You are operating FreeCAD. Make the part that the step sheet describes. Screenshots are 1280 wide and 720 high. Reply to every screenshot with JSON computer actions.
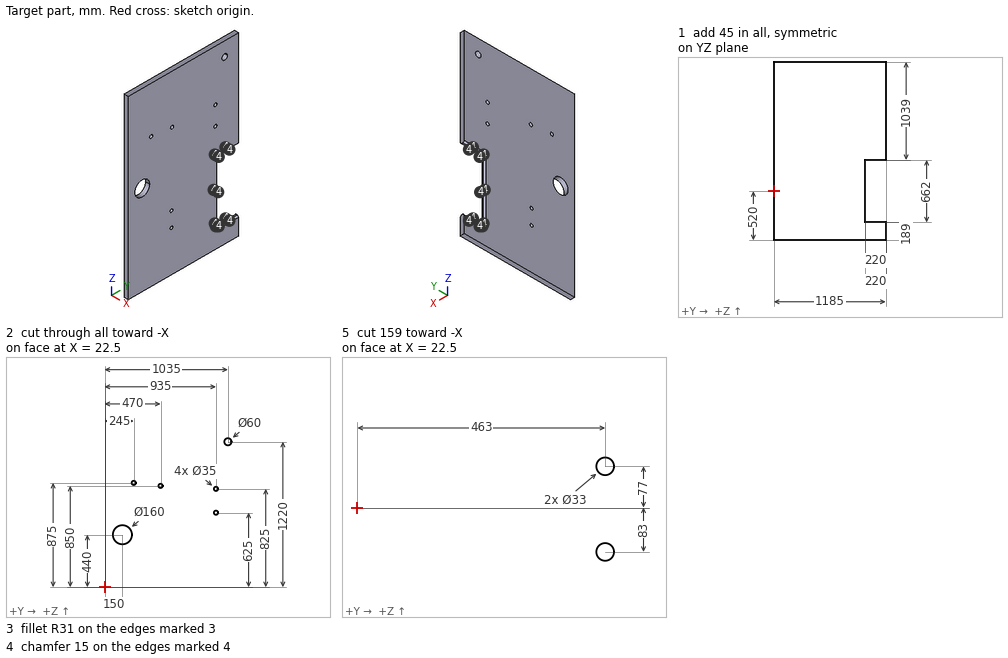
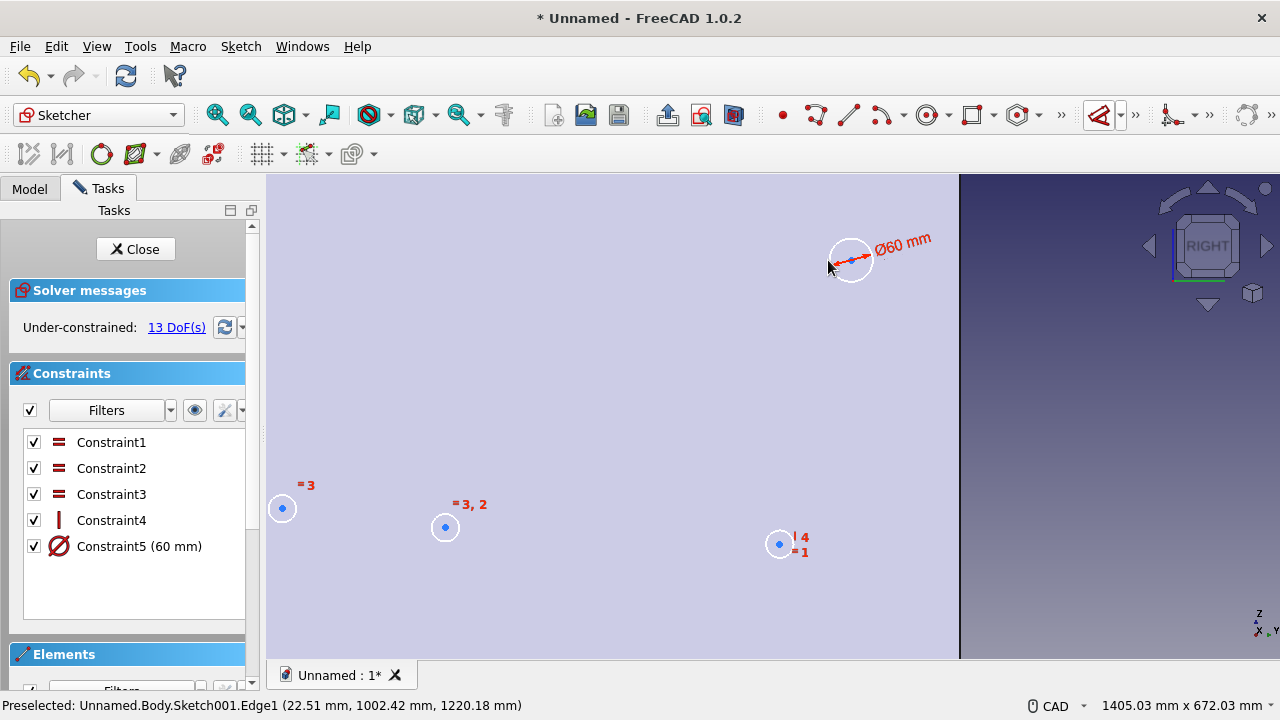
{"action": "scroll", "coordinate": [789, 534], "scroll_direction": "up", "scroll_amount": 3}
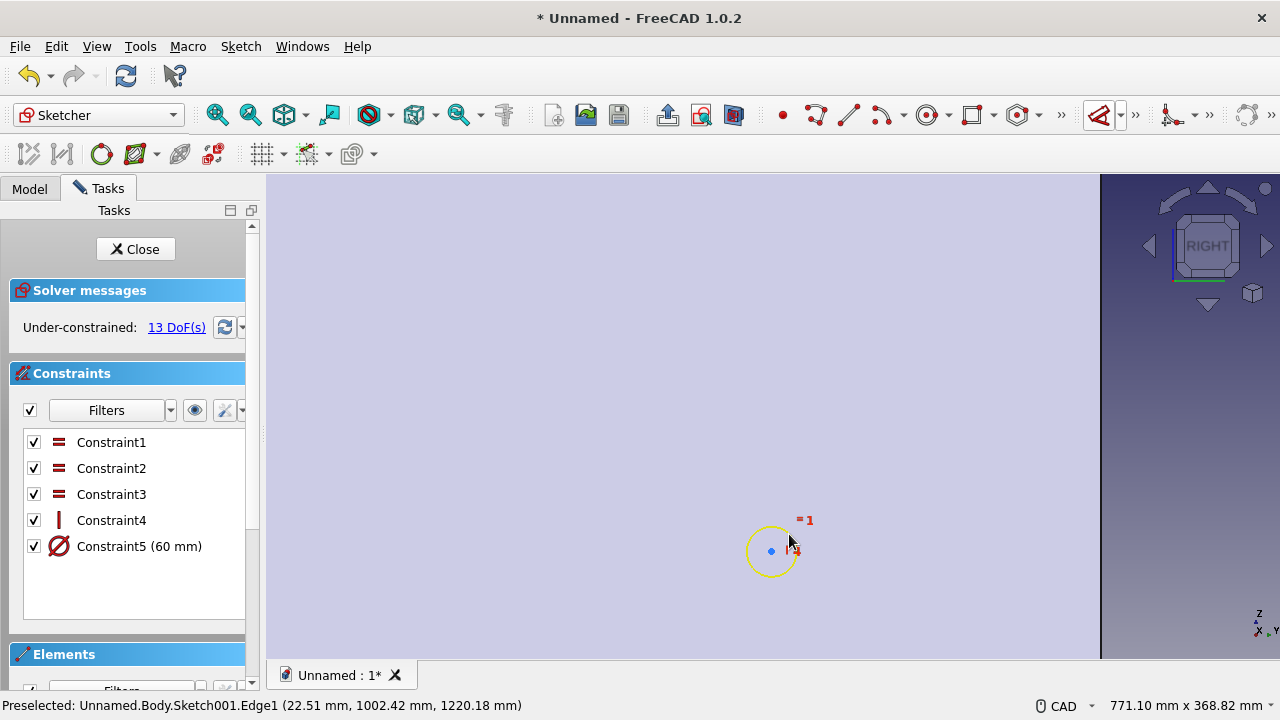
{"action": "left_click", "coordinate": [789, 534]}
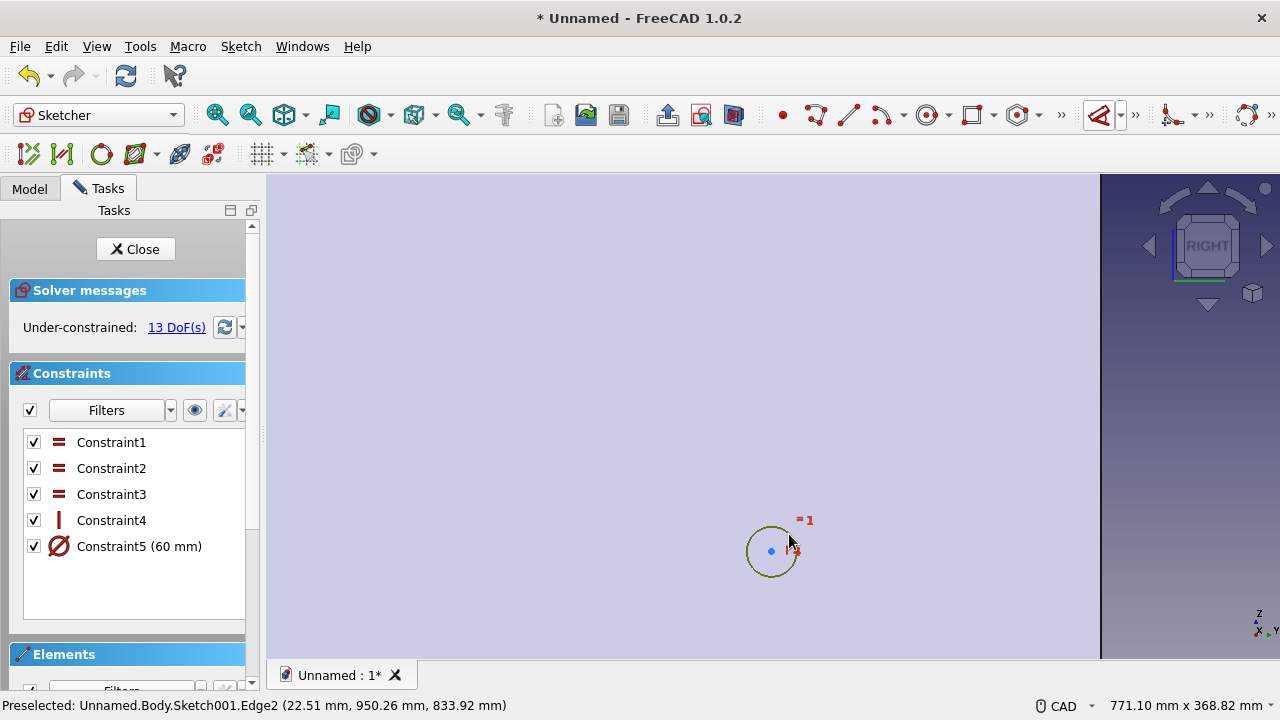
{"action": "left_click", "coordinate": [1120, 116]}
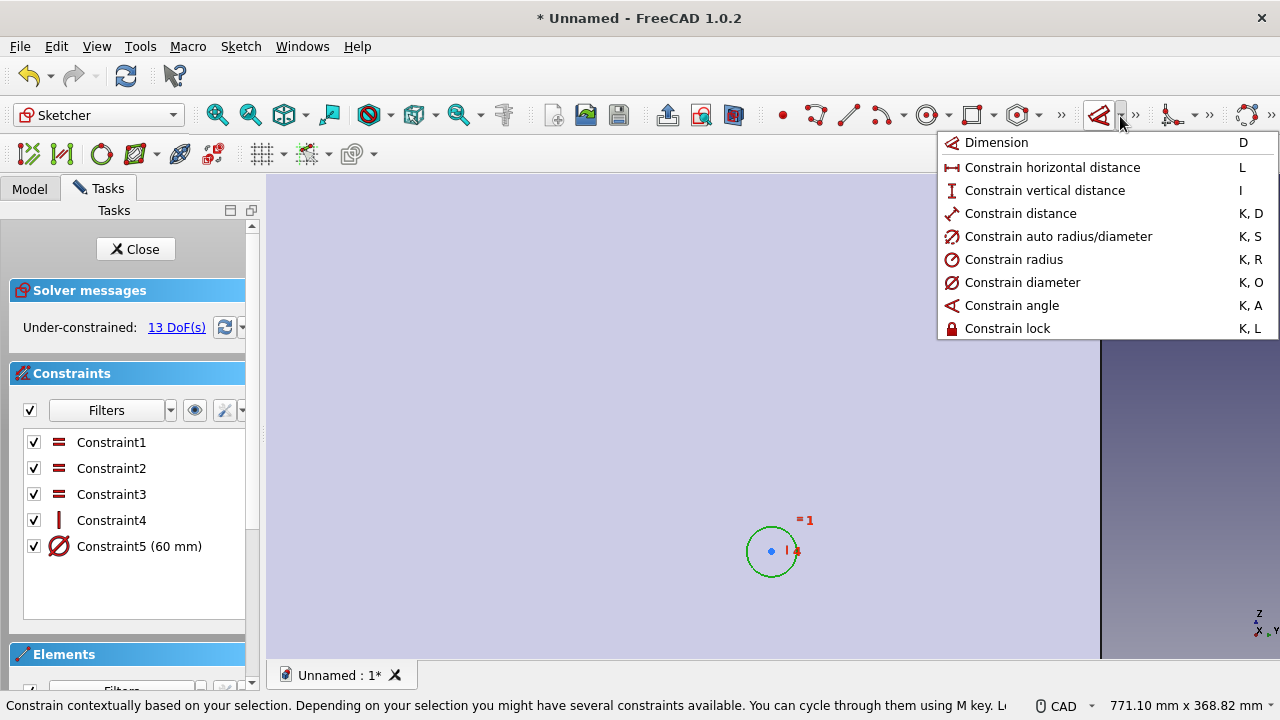
{"action": "left_click", "coordinate": [1108, 282]}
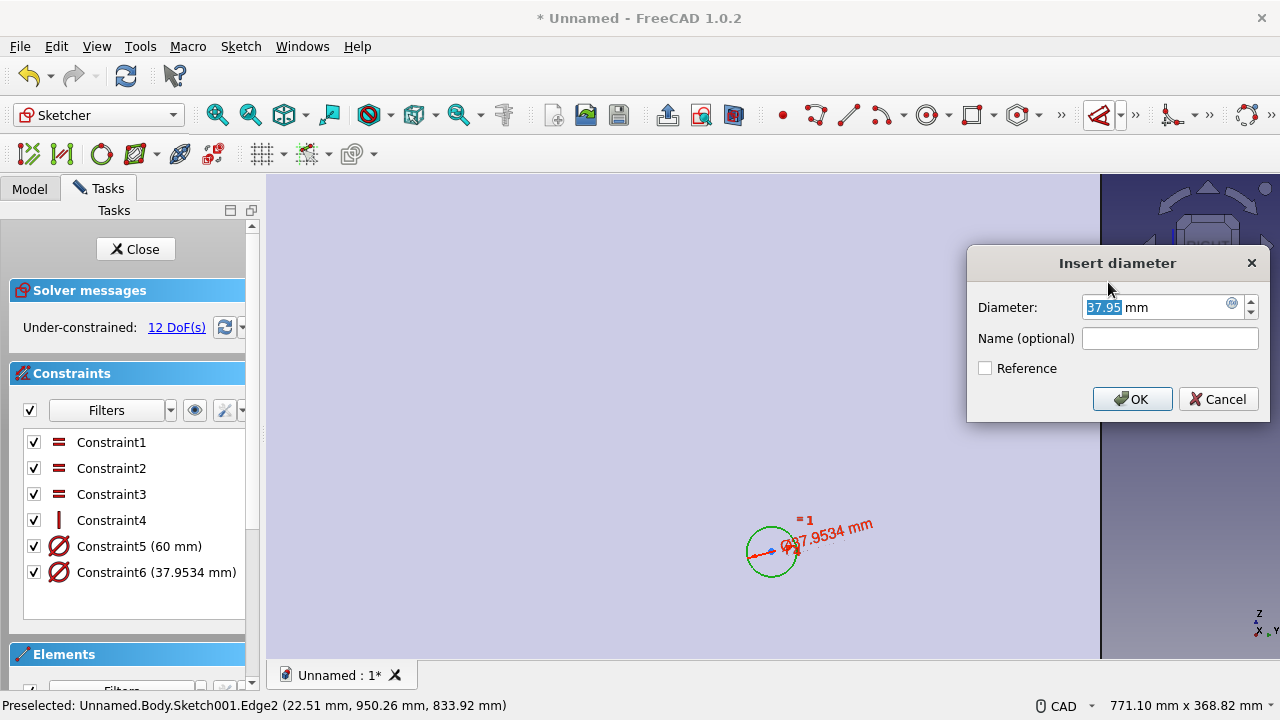
{"action": "type", "text": "35"}
{"action": "key", "text": "Return"}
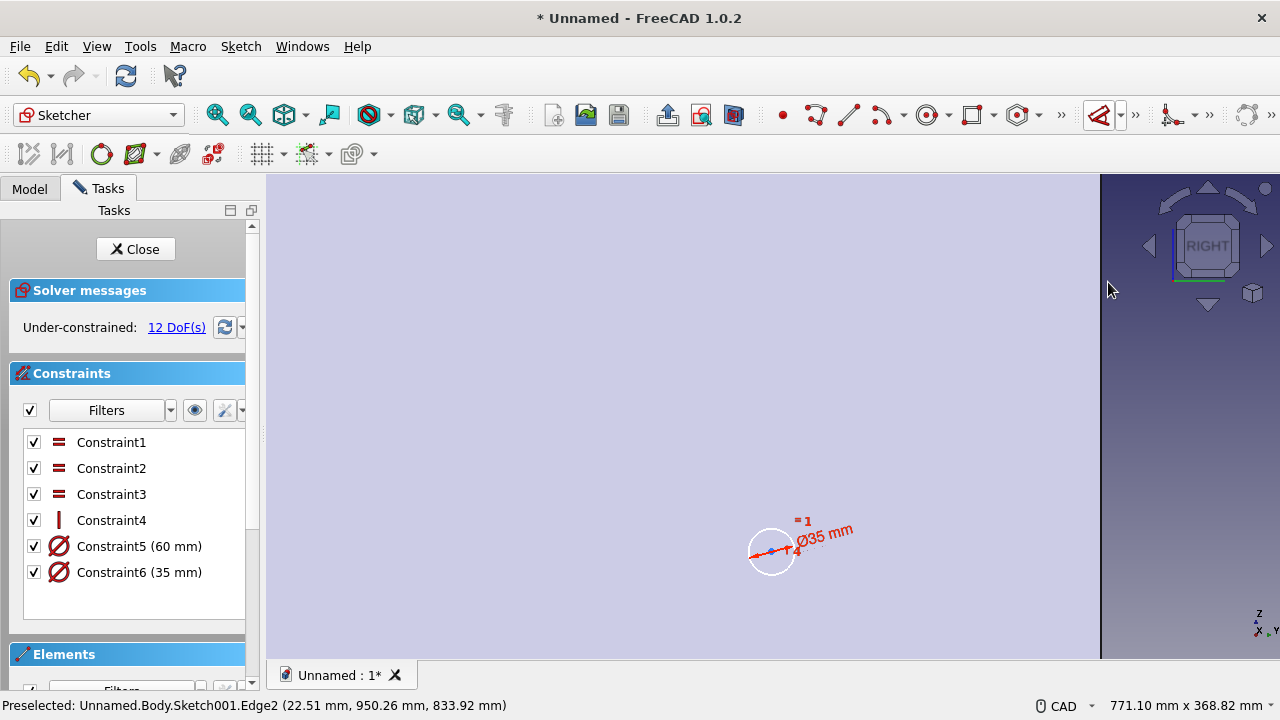
{"action": "scroll", "coordinate": [821, 316], "scroll_direction": "down", "scroll_amount": 8}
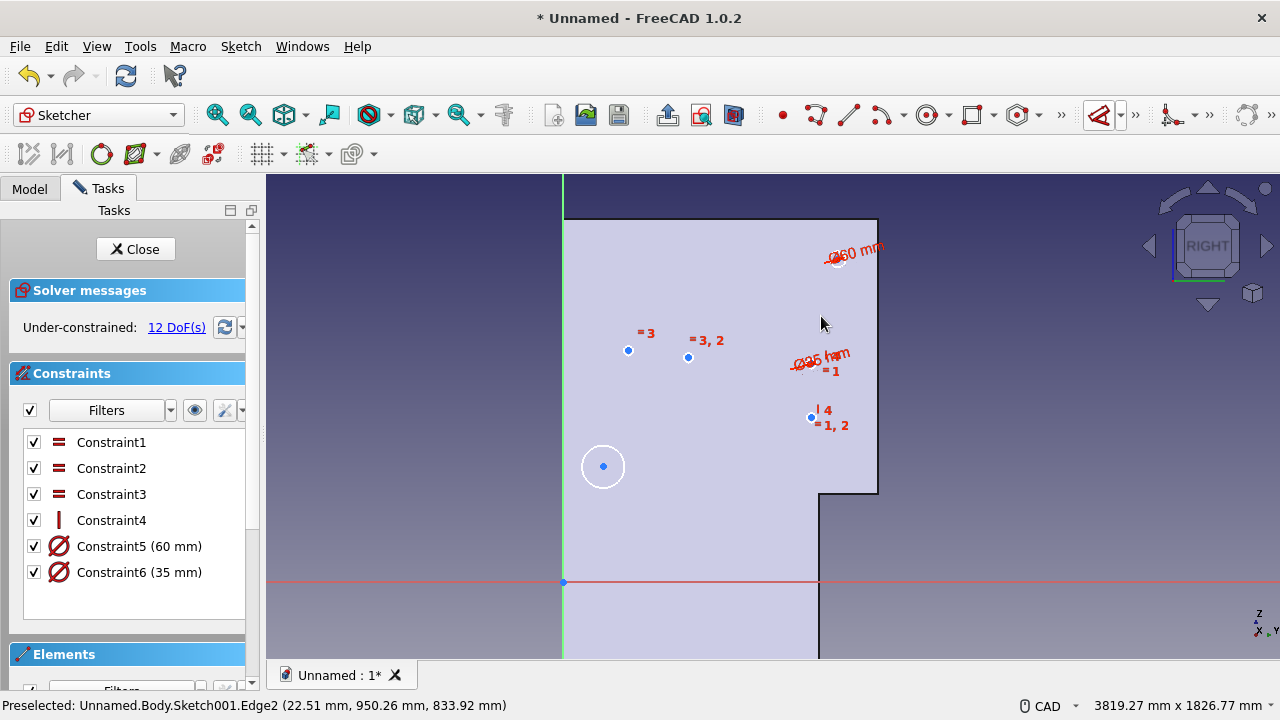
{"action": "left_click", "coordinate": [618, 452]}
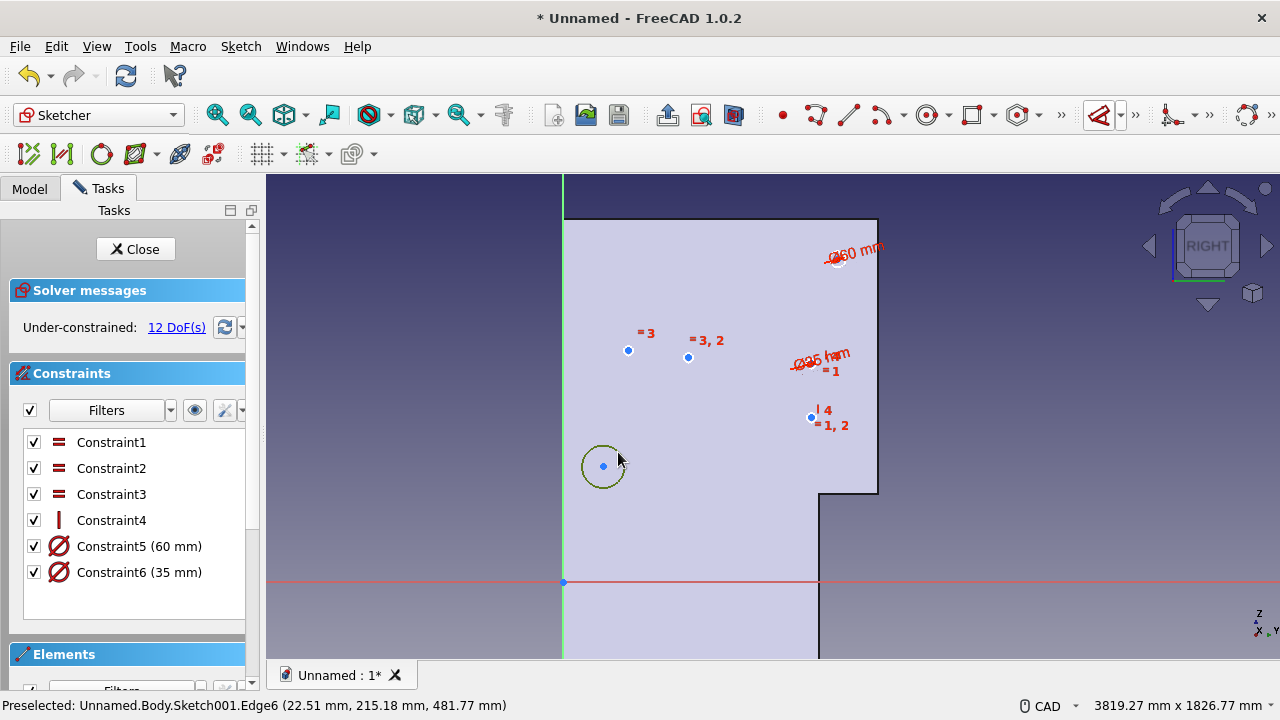
{"action": "left_click", "coordinate": [1120, 116]}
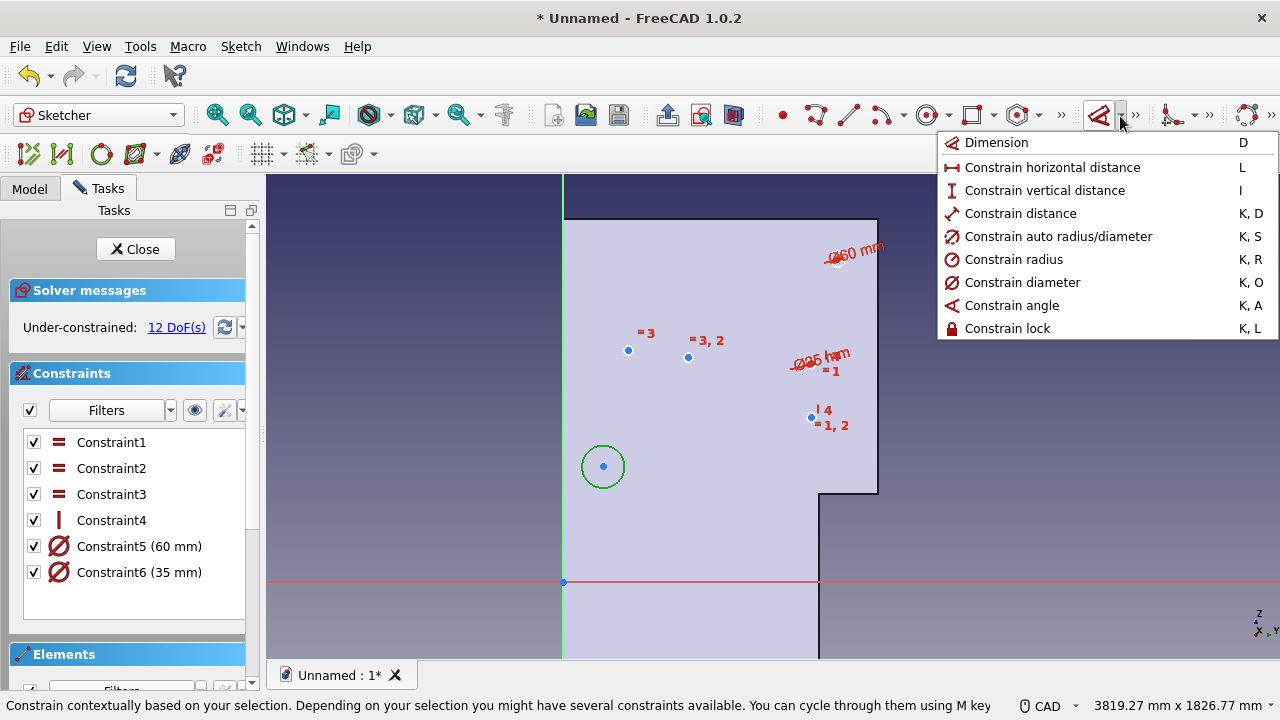
{"action": "left_click", "coordinate": [1108, 282]}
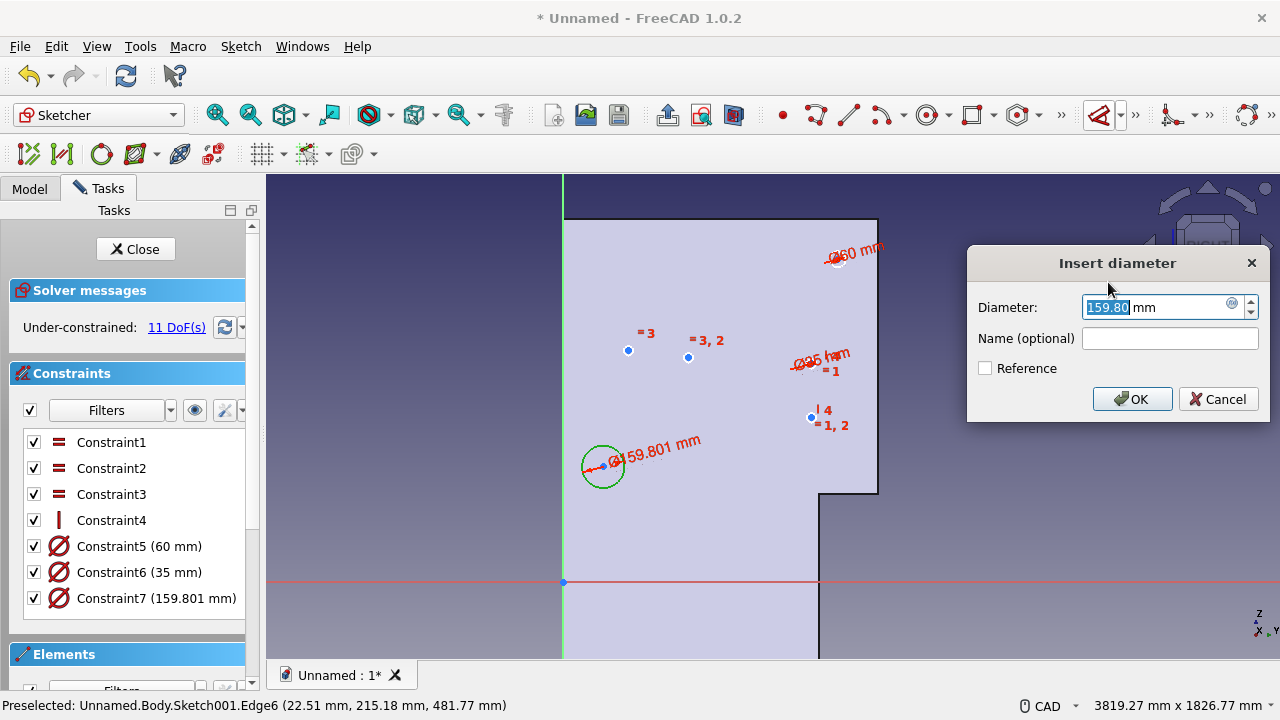
{"action": "type", "text": "160"}
{"action": "key", "text": "Return"}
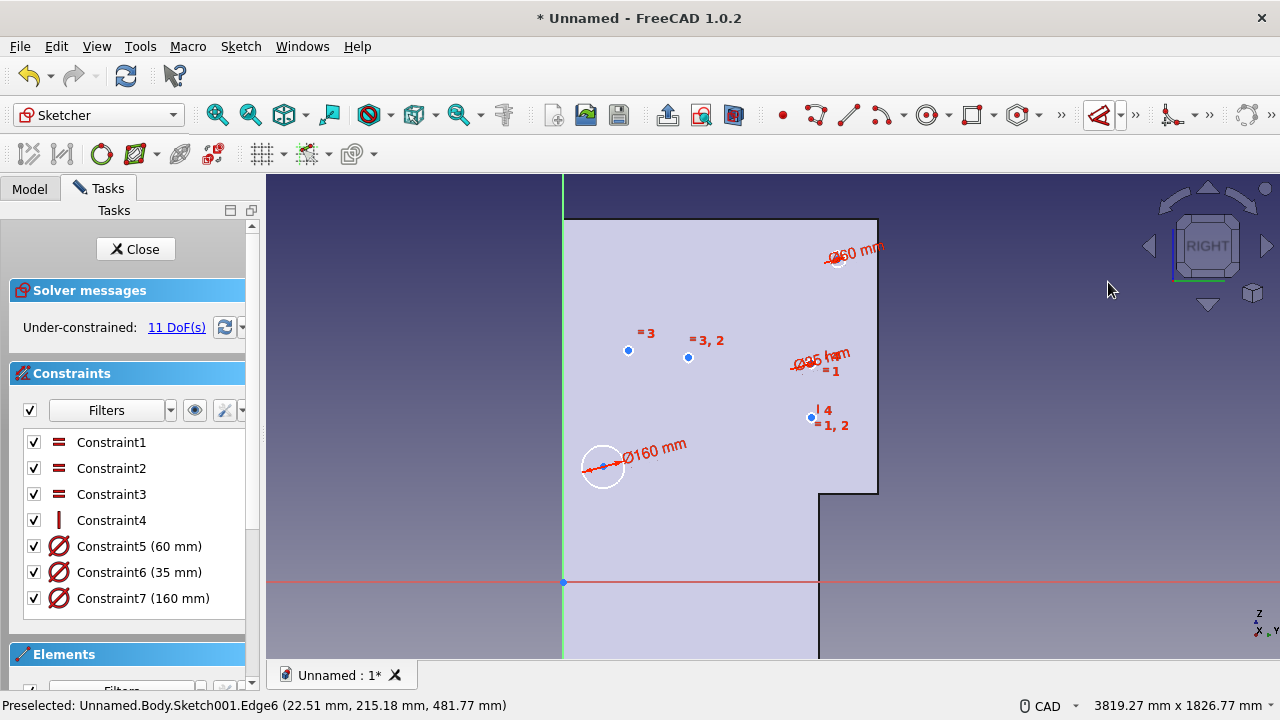
{"action": "left_click", "coordinate": [812, 364]}